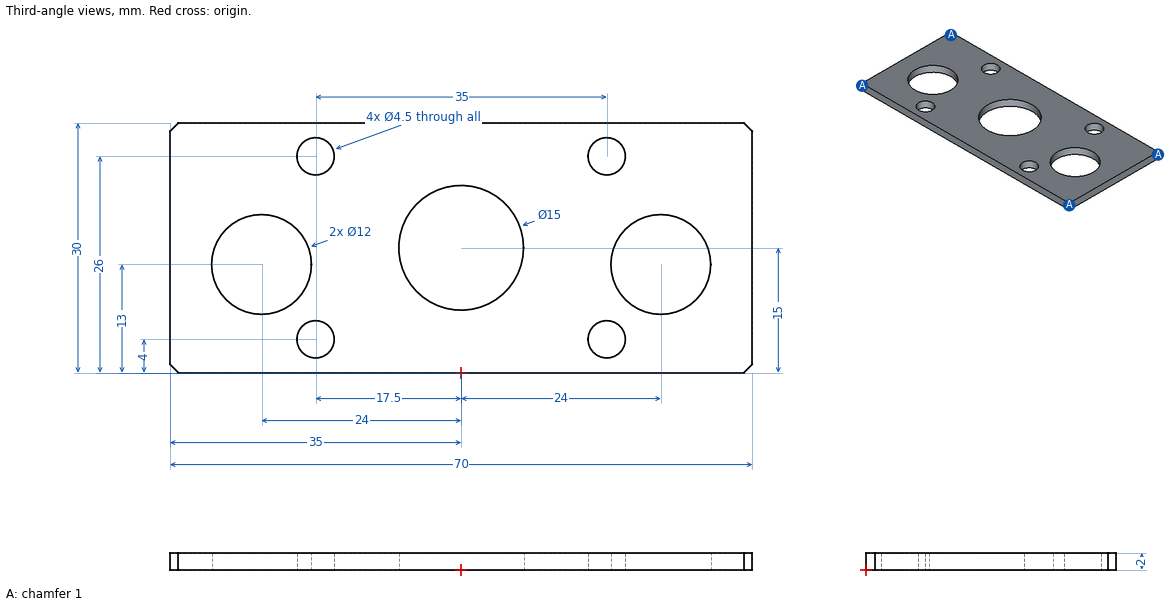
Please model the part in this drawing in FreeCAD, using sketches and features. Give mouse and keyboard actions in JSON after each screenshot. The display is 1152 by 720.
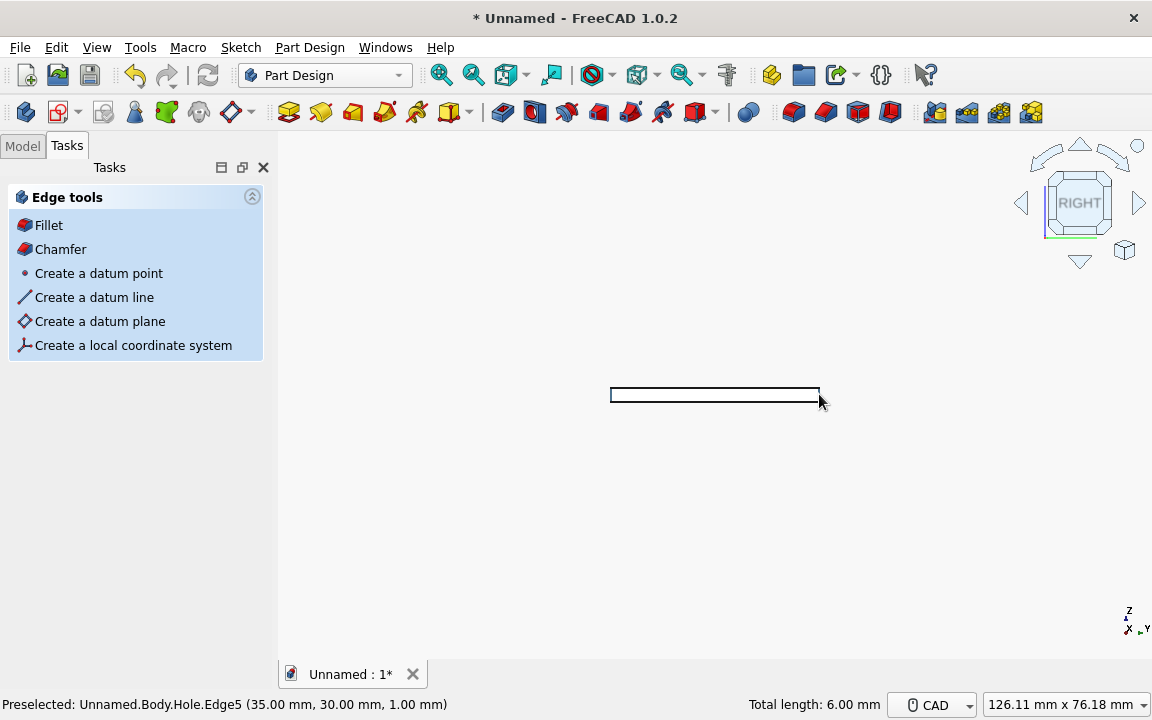
{"action": "scroll", "coordinate": [819, 394], "scroll_direction": "up", "scroll_amount": 6}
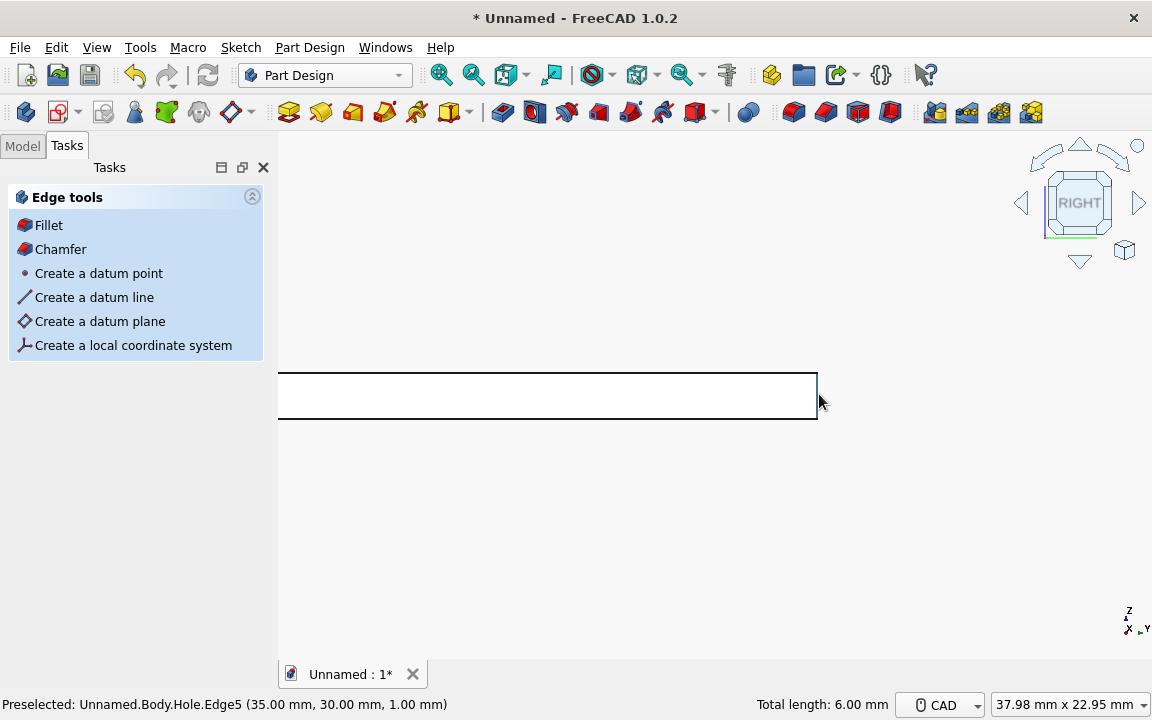
{"action": "left_click", "coordinate": [442, 76]}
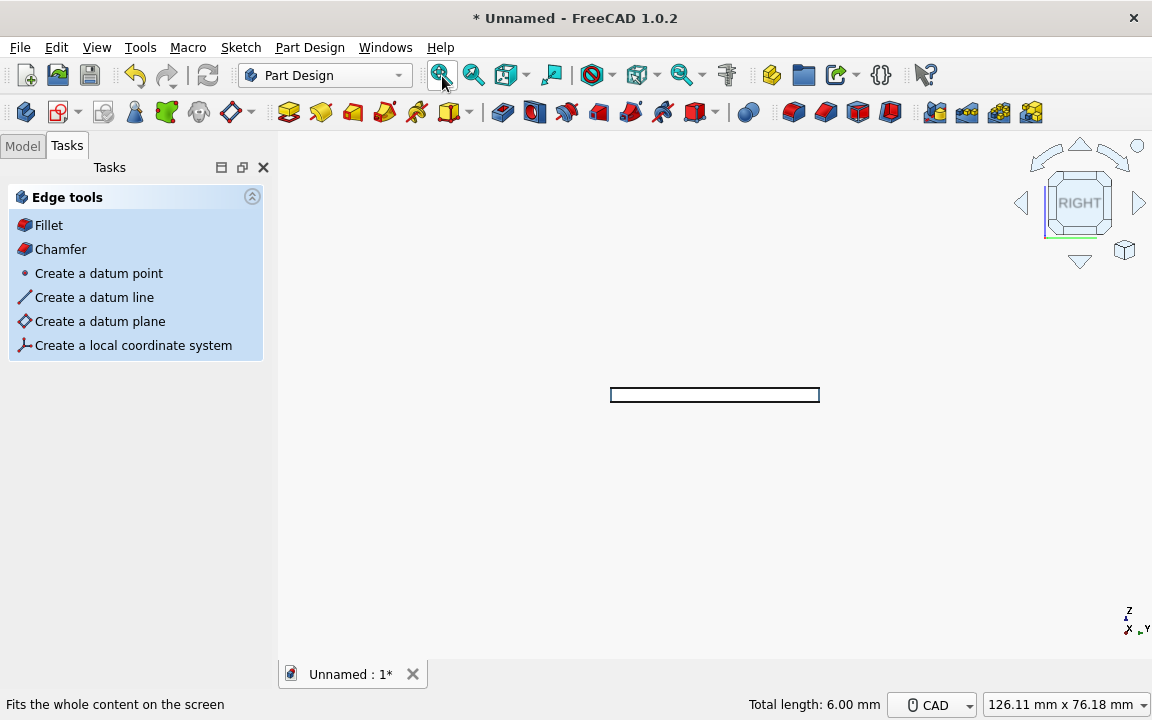
{"action": "key", "text": "5"}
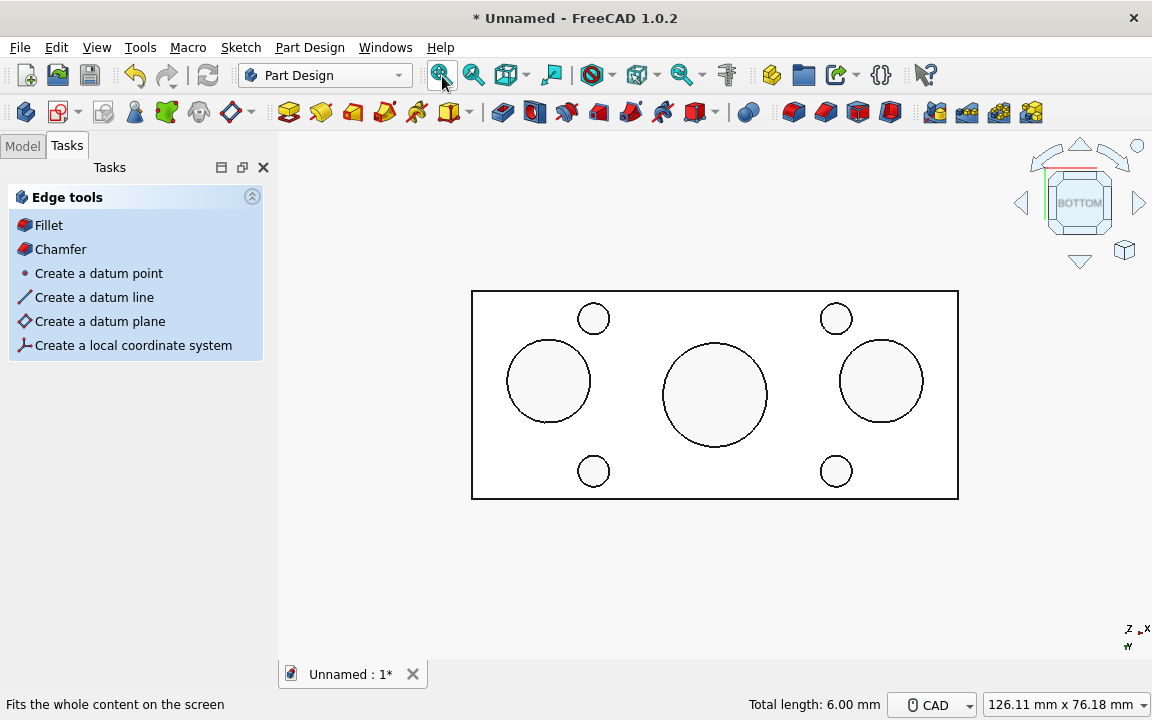
{"action": "scroll", "coordinate": [472, 498], "scroll_direction": "up", "scroll_amount": 6}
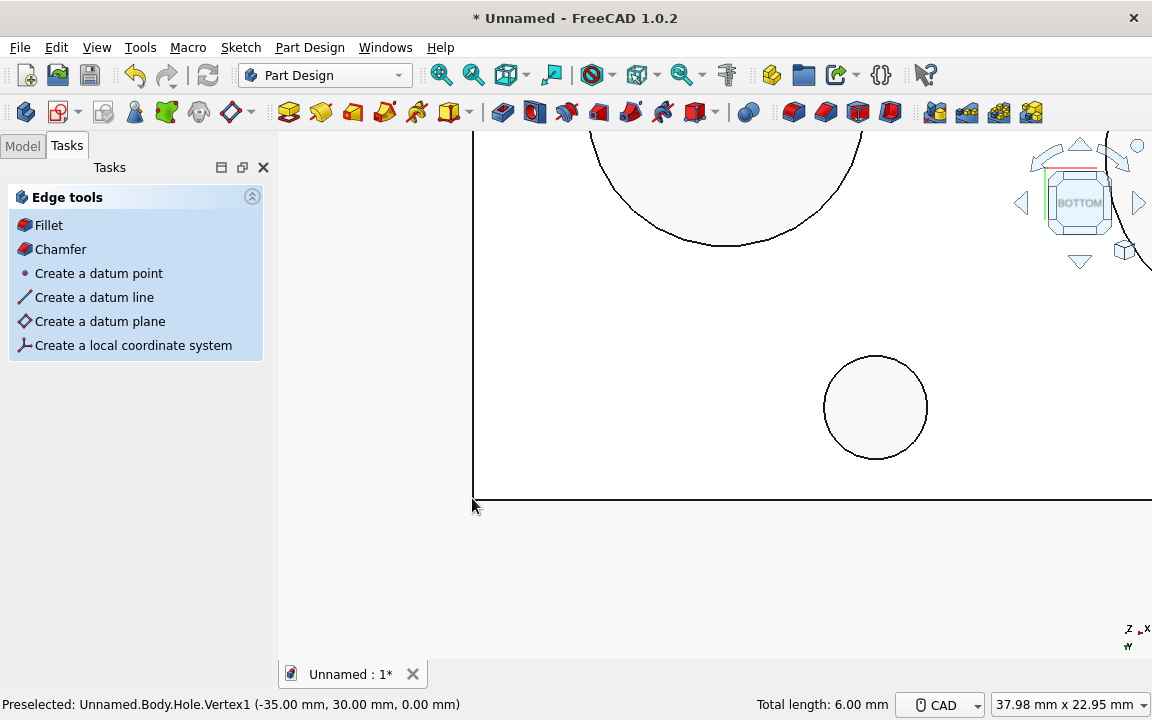
{"action": "left_click", "coordinate": [442, 76]}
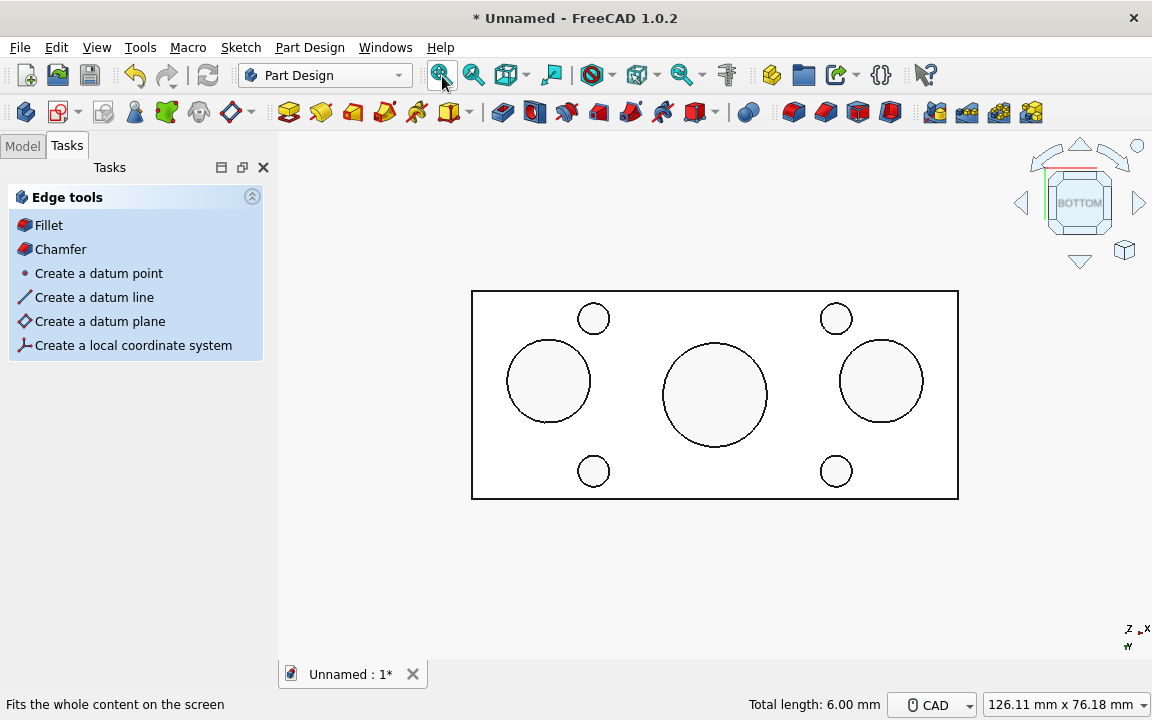
{"action": "key", "text": "4"}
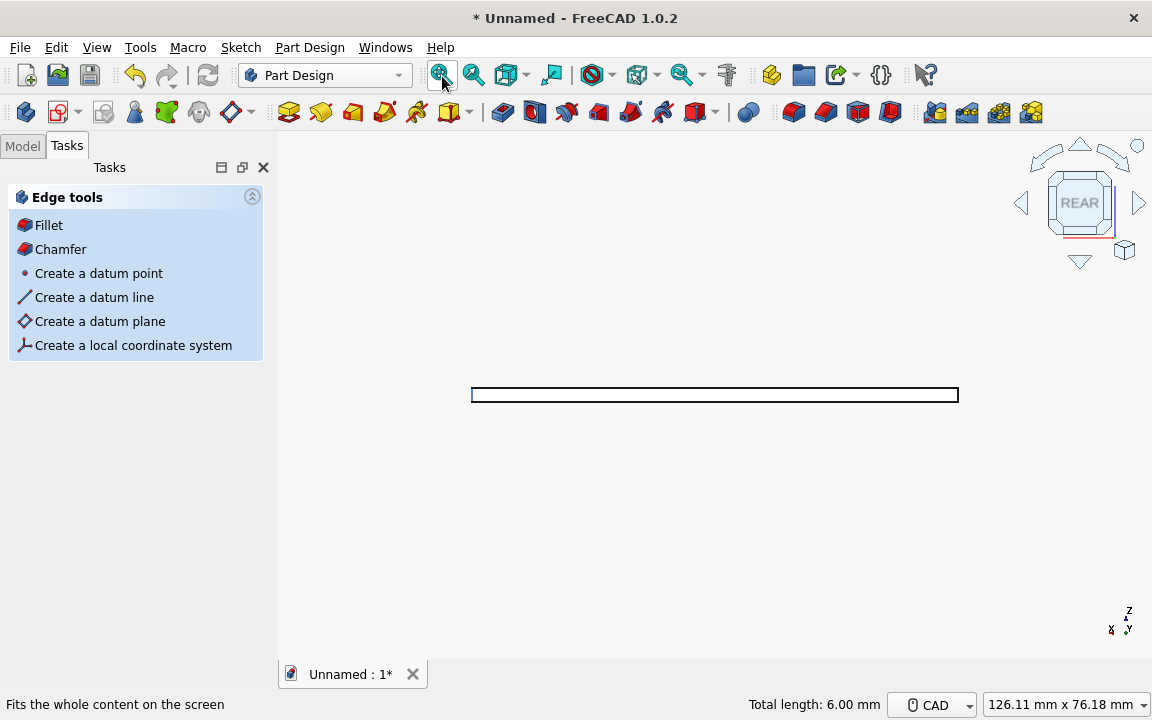
{"action": "left_click", "coordinate": [958, 394], "text": "ctrl"}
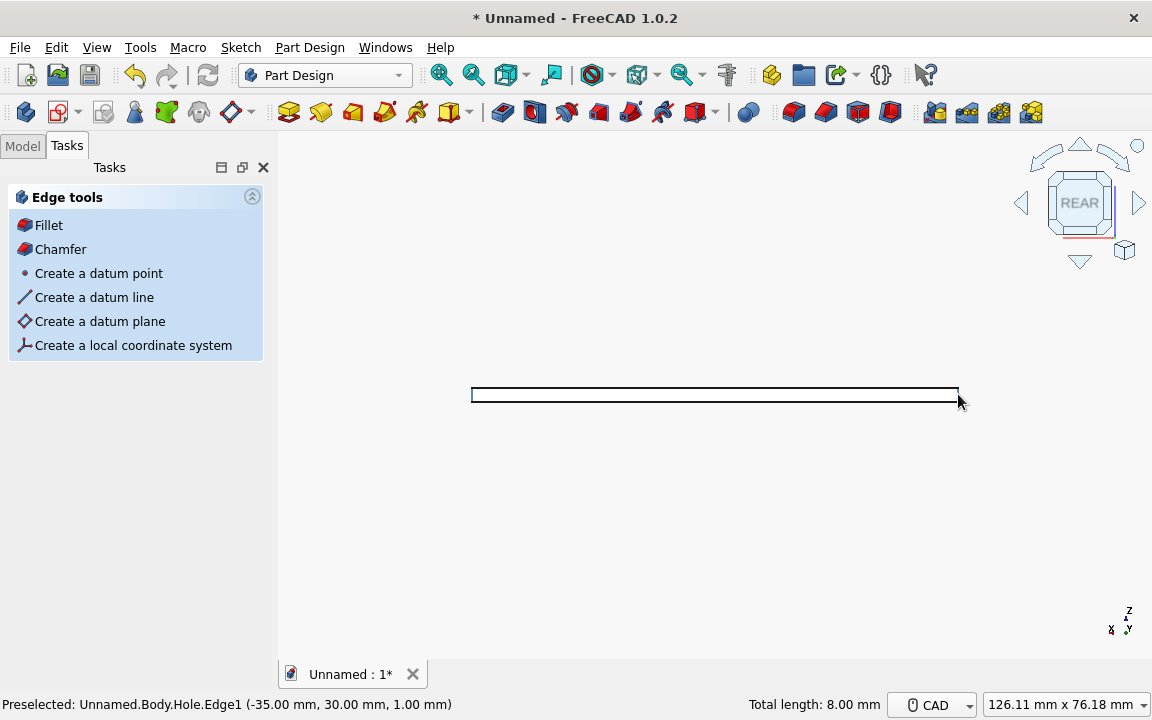
{"action": "left_click", "coordinate": [826, 112]}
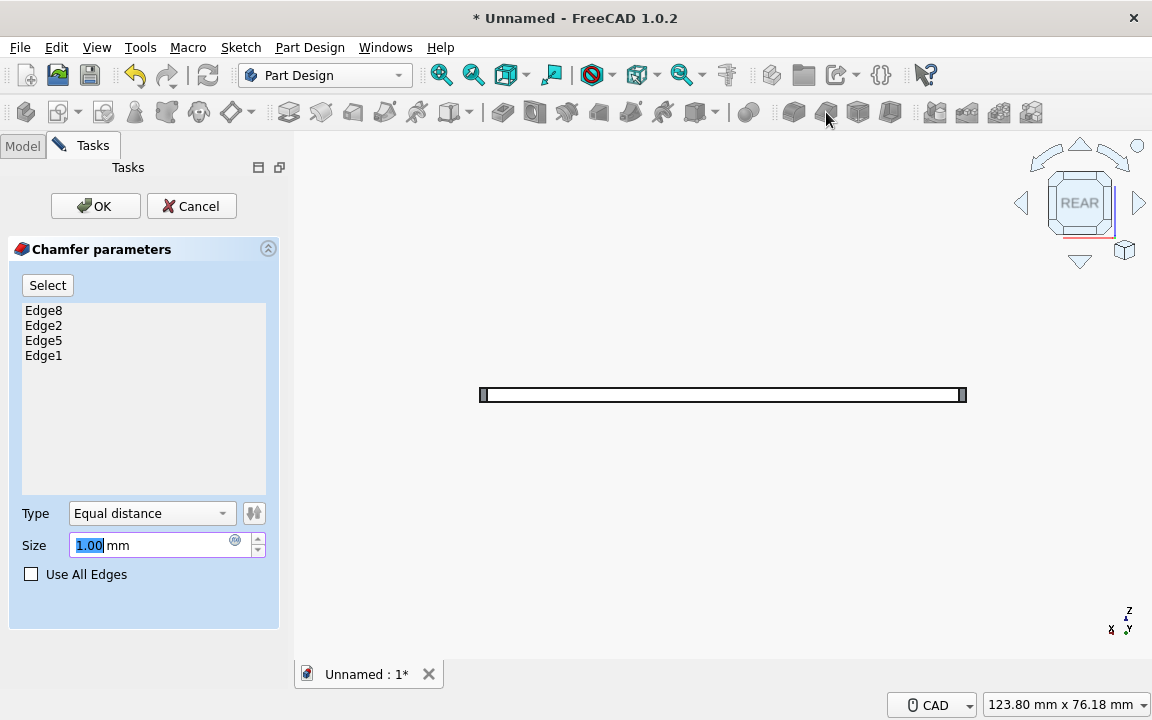
{"action": "type", "text": "1"}
{"action": "key", "text": "Tab"}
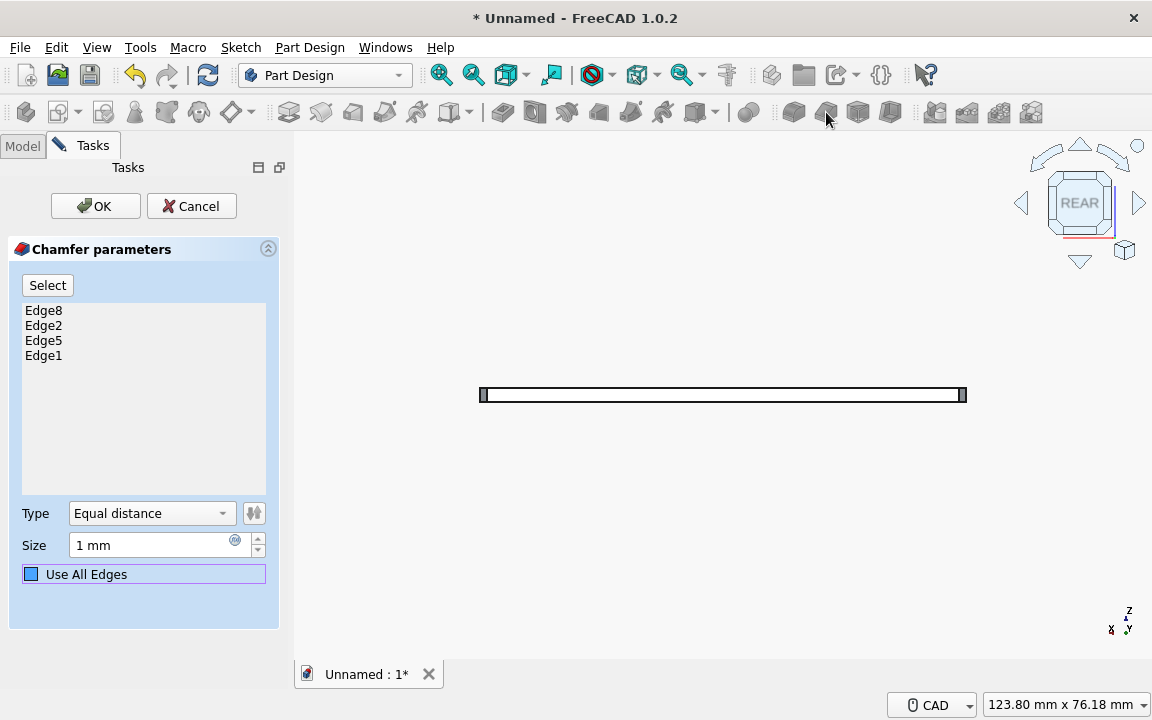
{"action": "left_click", "coordinate": [96, 206]}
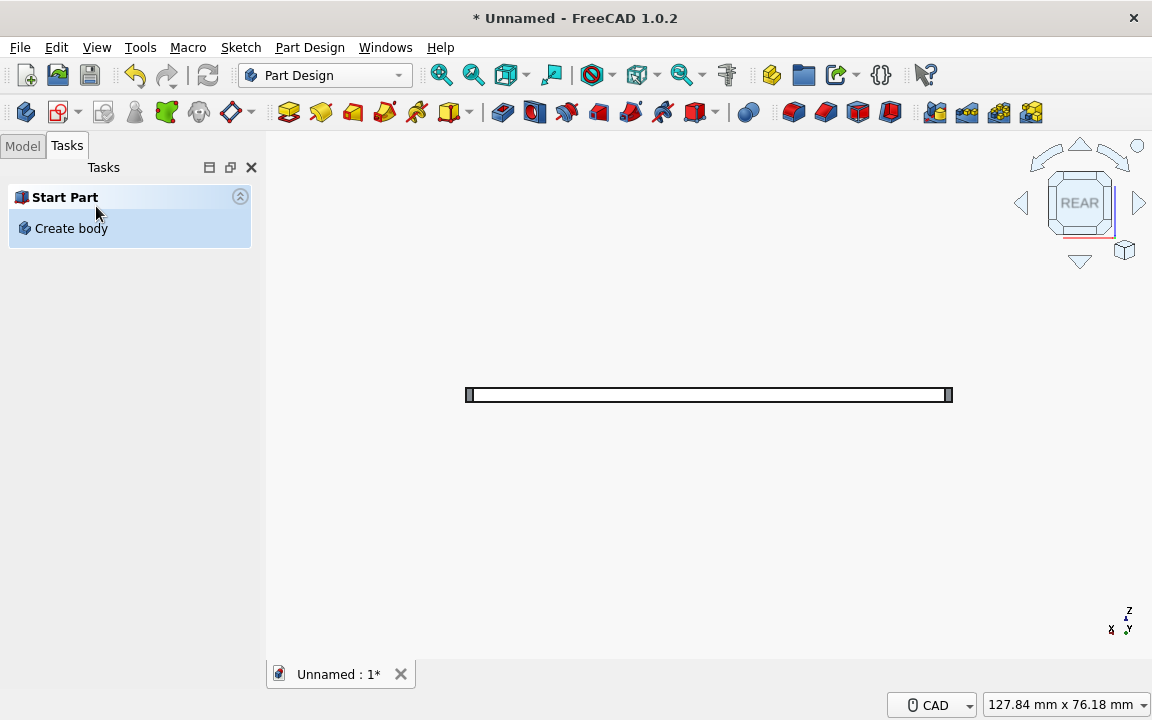
{"action": "key", "text": "0"}